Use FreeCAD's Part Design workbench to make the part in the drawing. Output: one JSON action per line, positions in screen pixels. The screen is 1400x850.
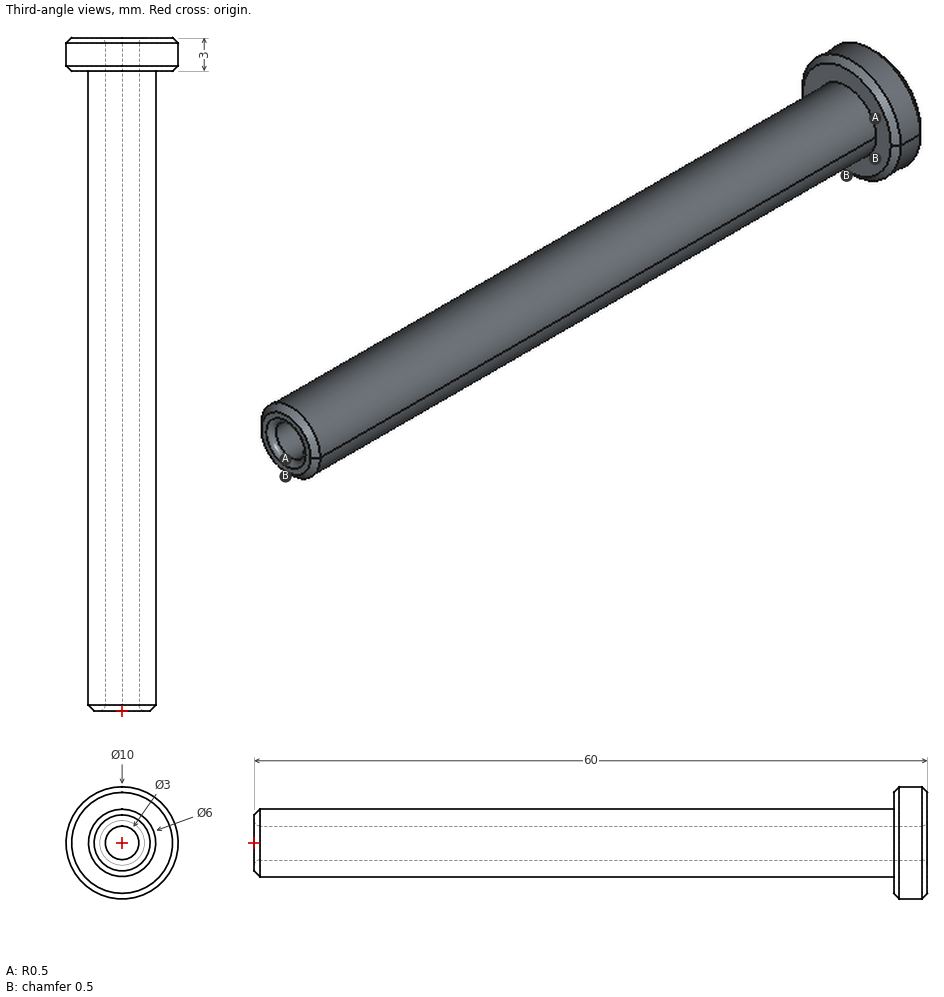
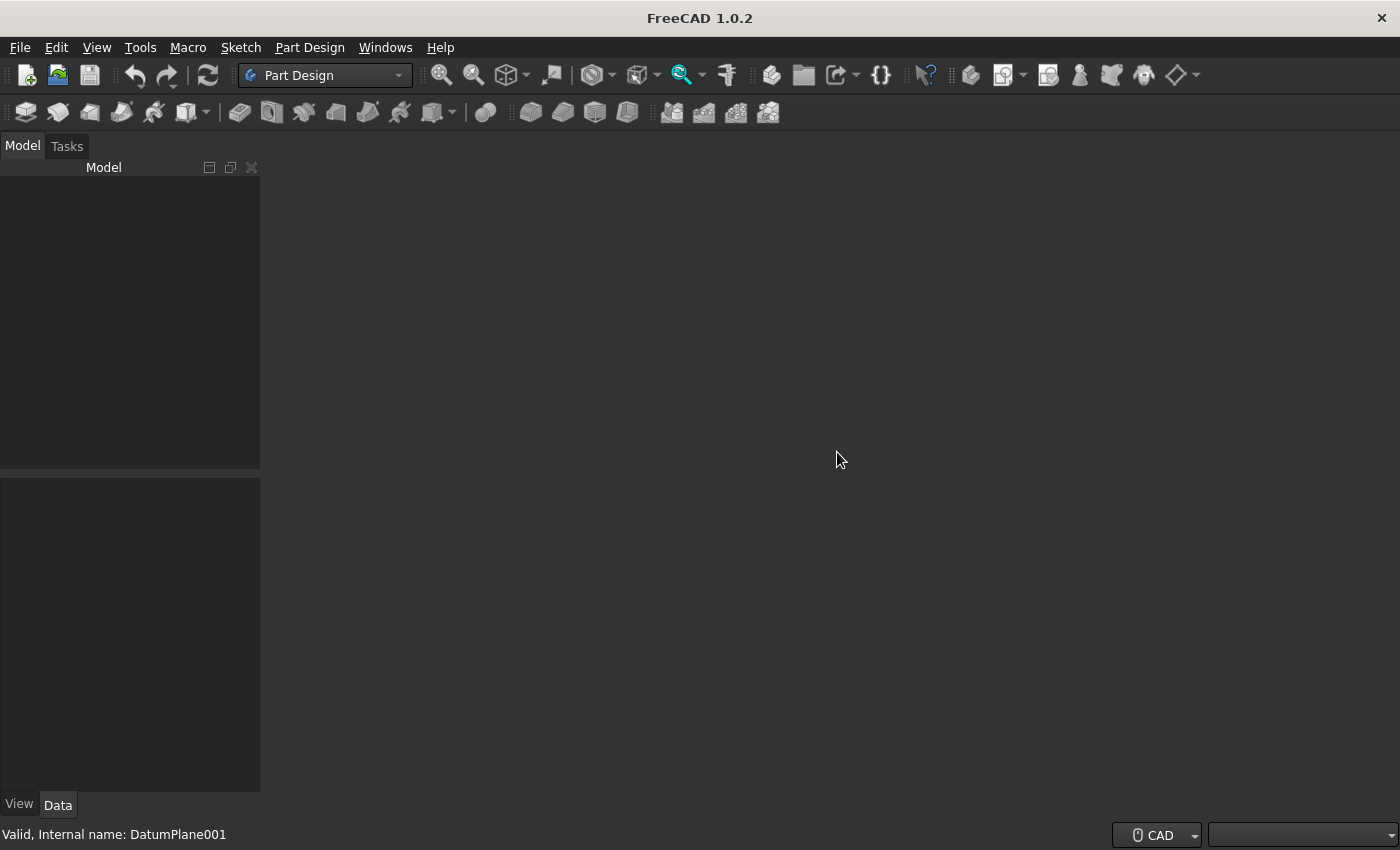
{"action": "key", "text": "ctrl+n"}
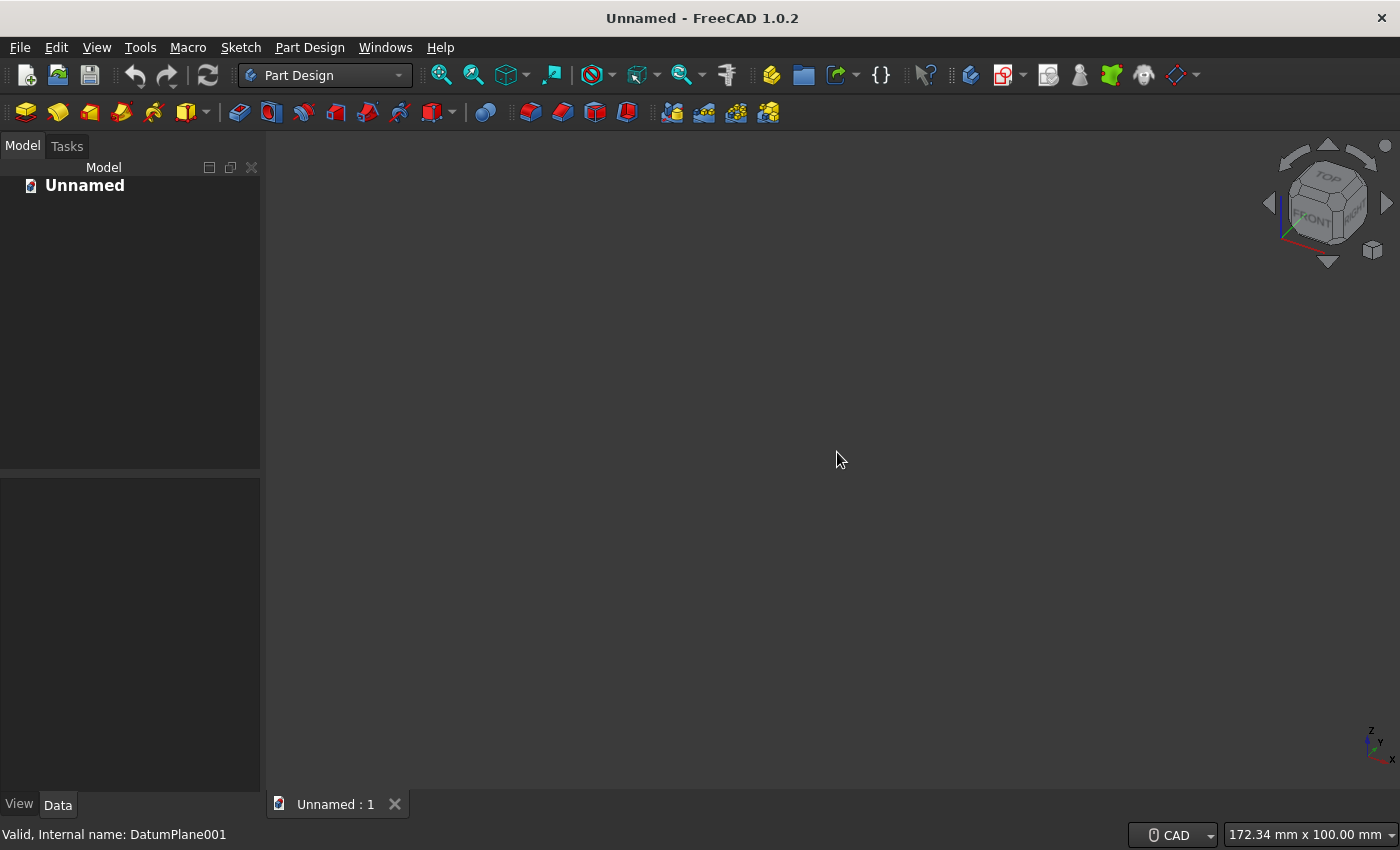
{"action": "left_click", "coordinate": [1004, 76]}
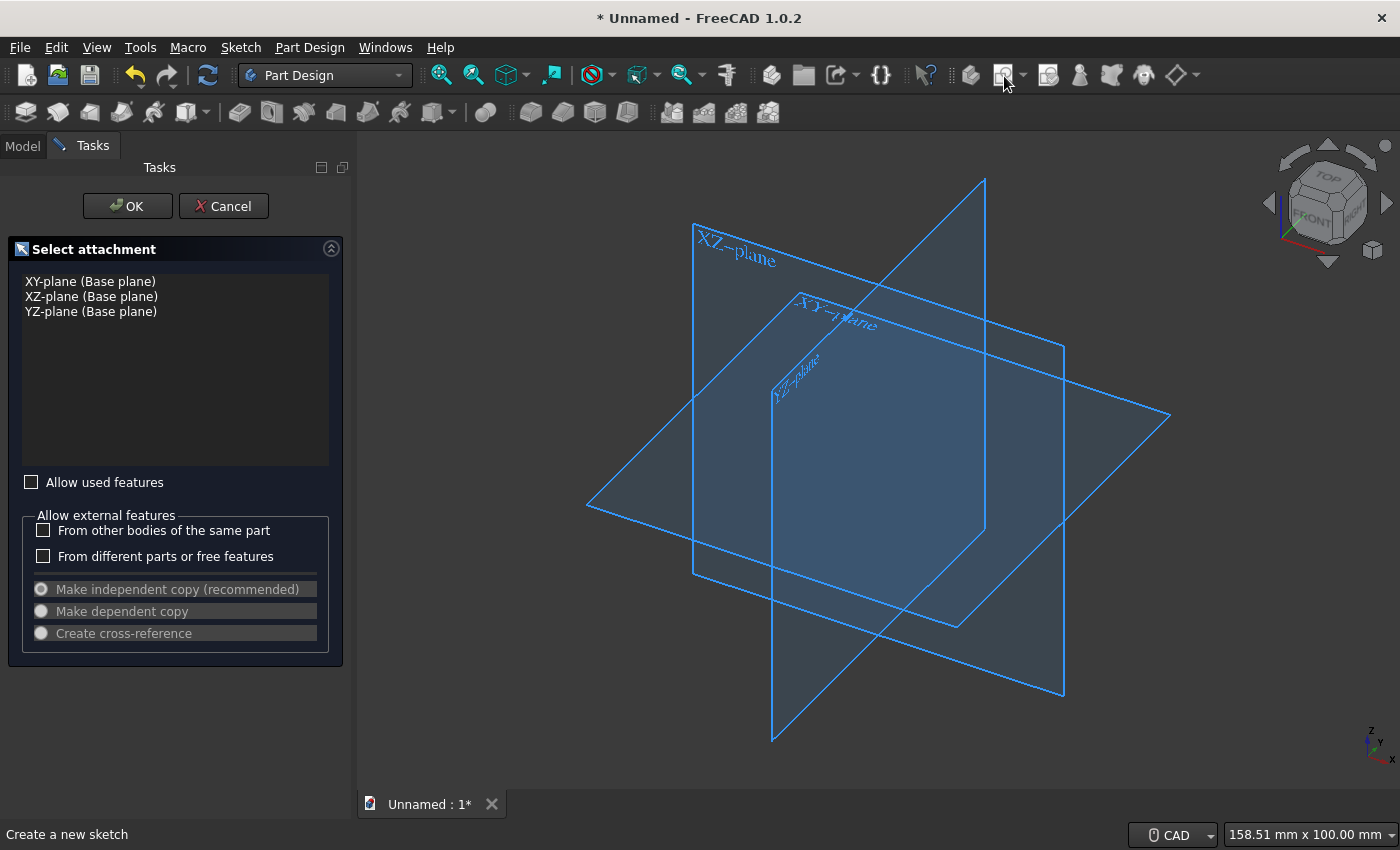
{"action": "left_click", "coordinate": [82, 296]}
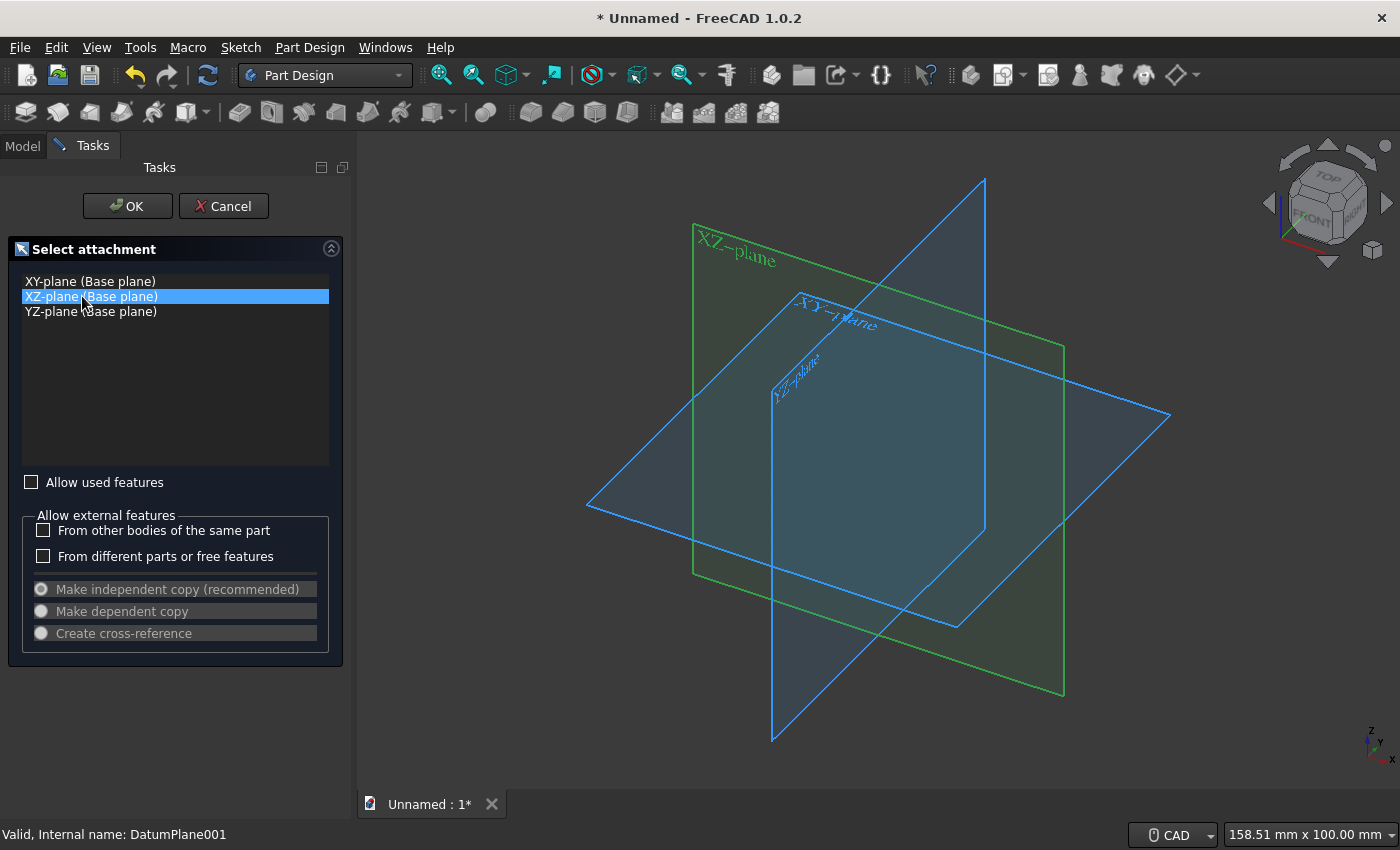
{"action": "left_click", "coordinate": [128, 206]}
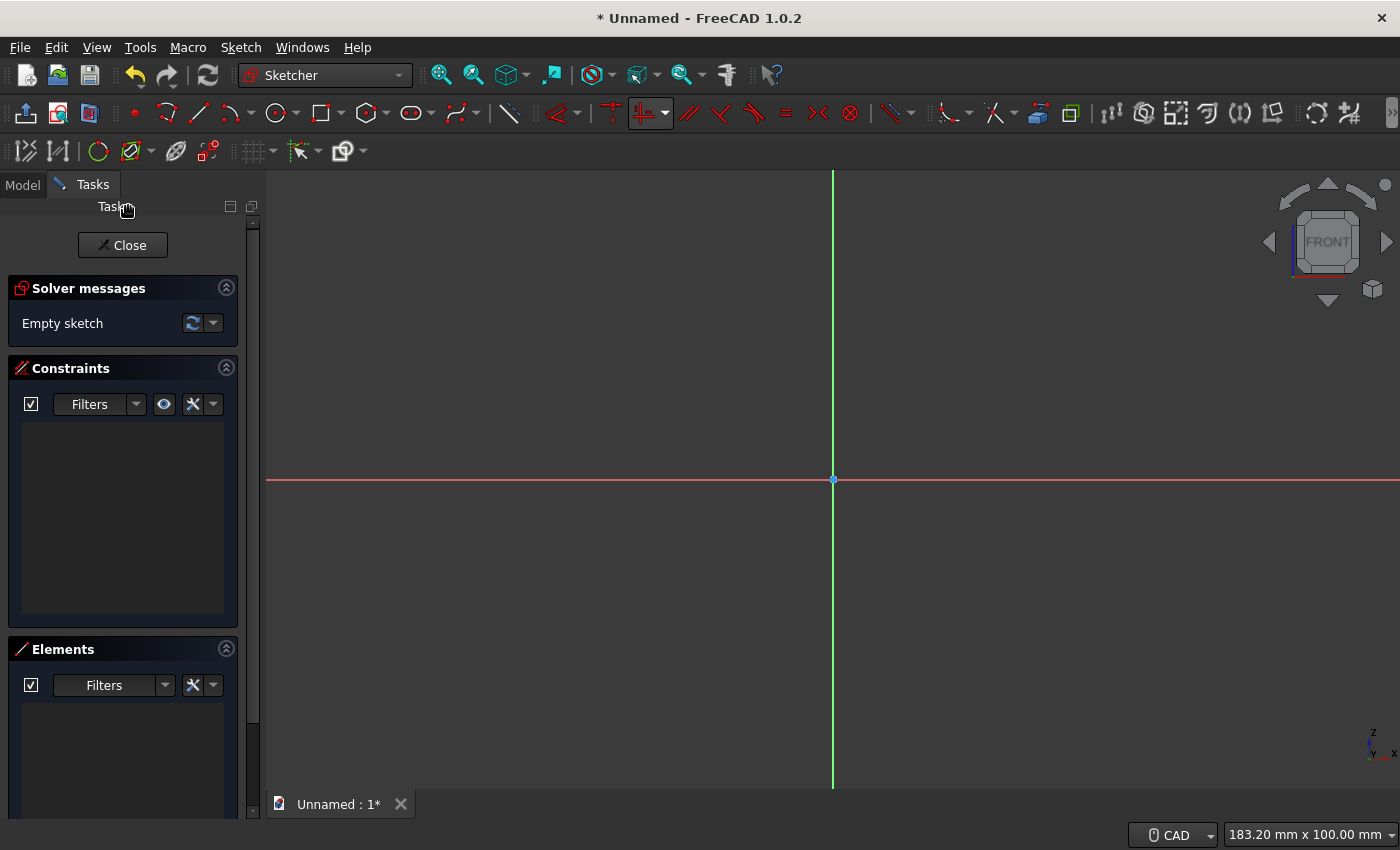
{"action": "scroll", "coordinate": [840, 480], "scroll_direction": "up", "scroll_amount": 12}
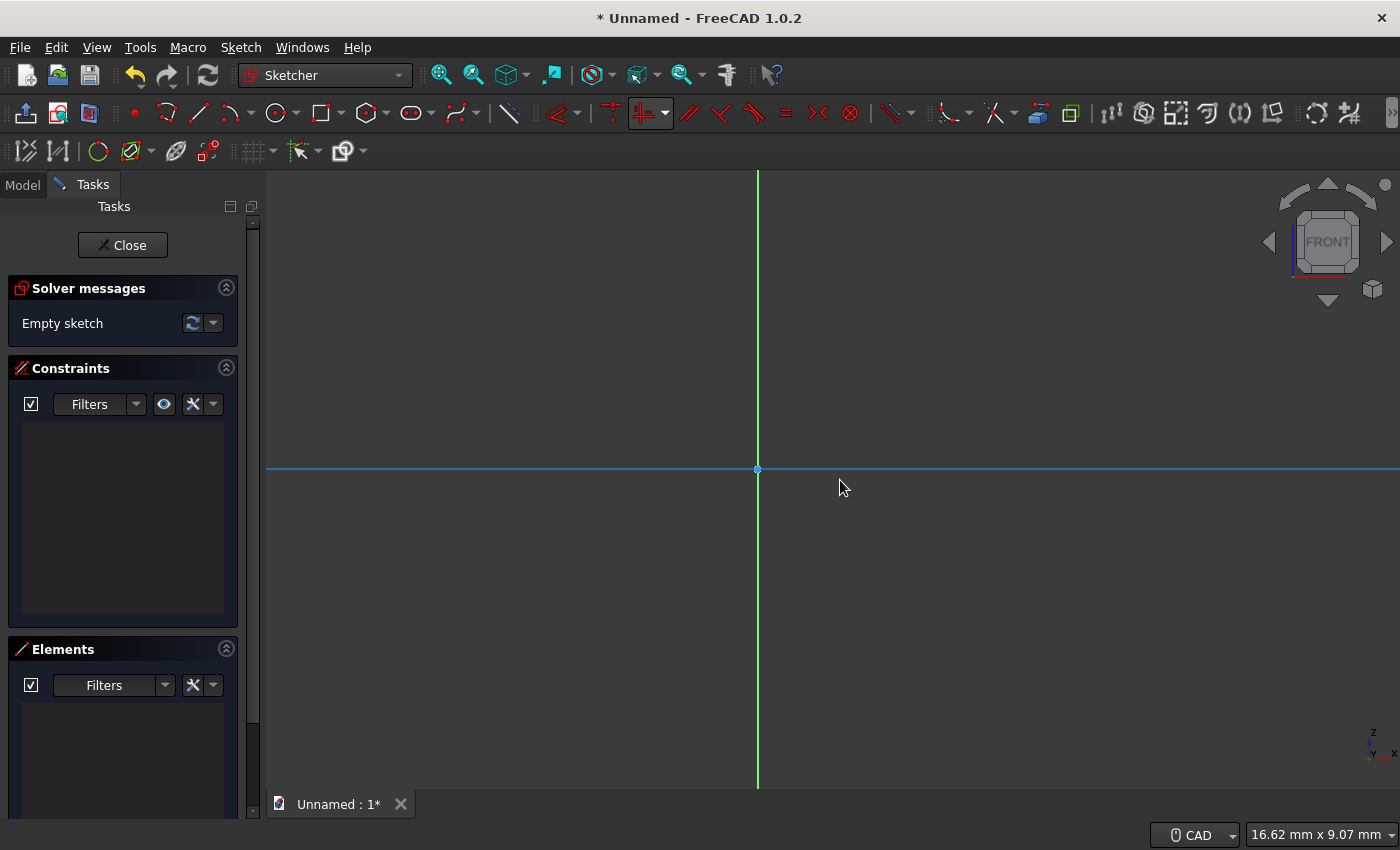
{"action": "key", "text": "g c"}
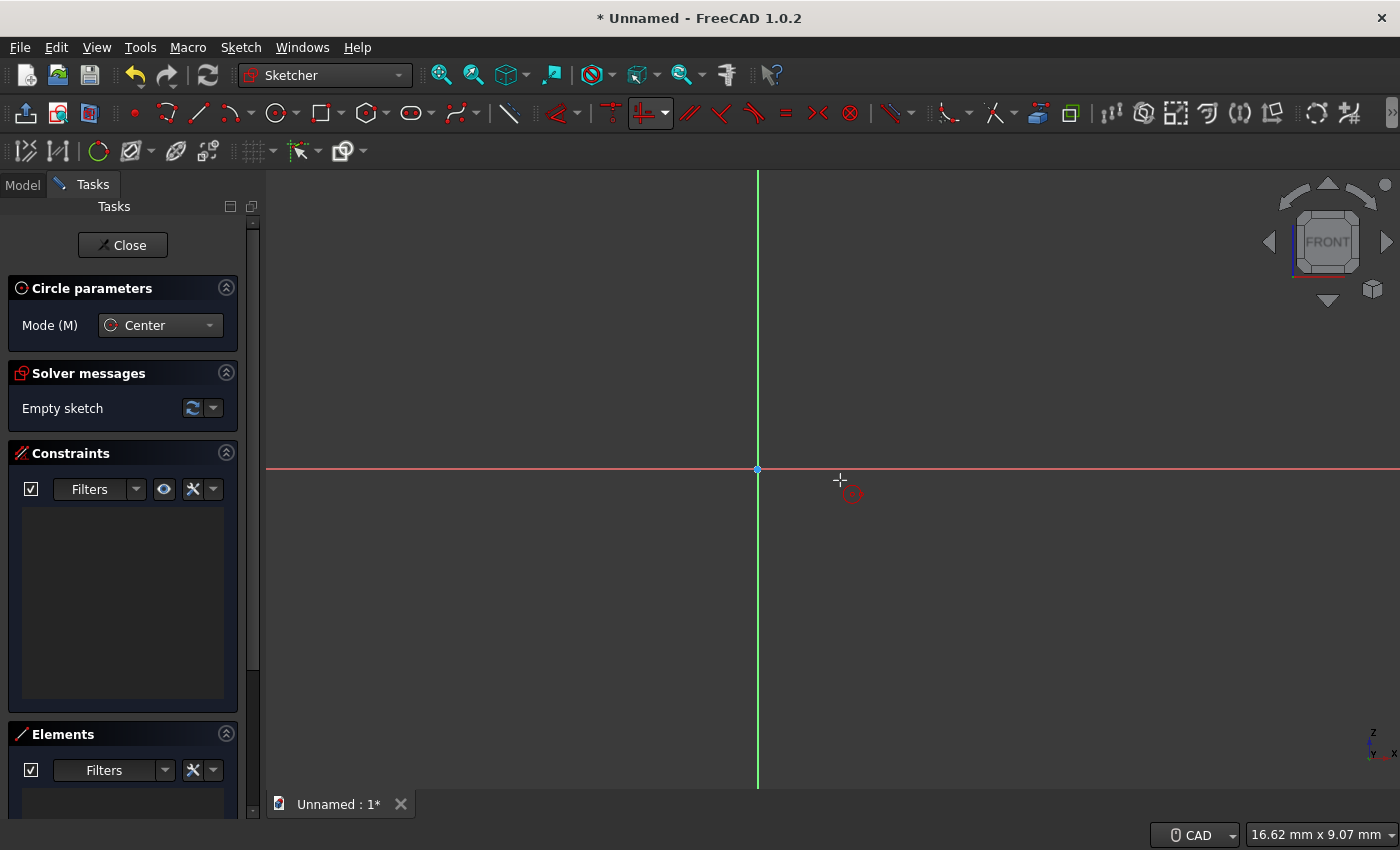
{"action": "left_click", "coordinate": [758, 469]}
{"action": "mouse_move", "coordinate": [903, 325]}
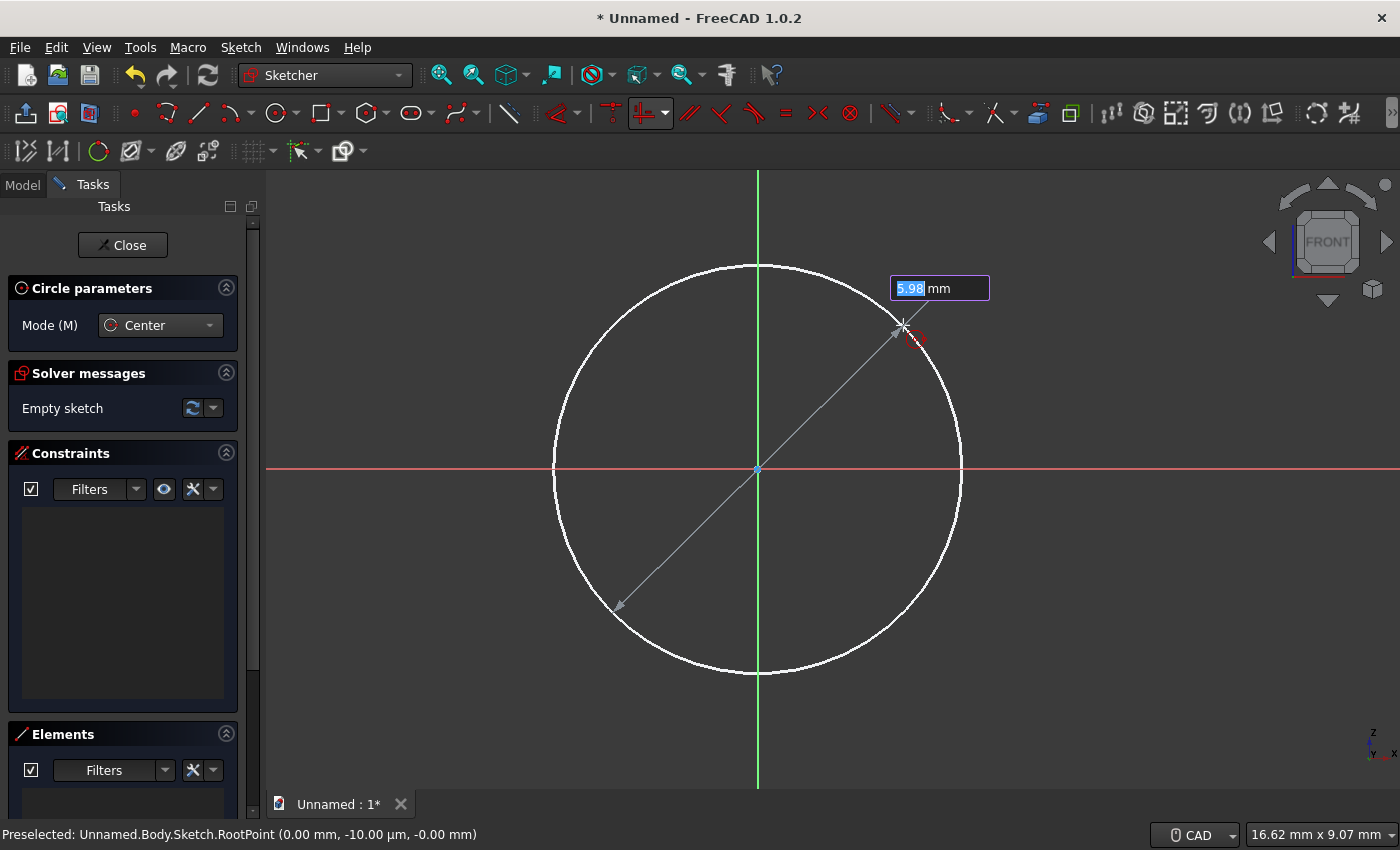
{"action": "type", "text": "6"}
{"action": "key", "text": "Return"}